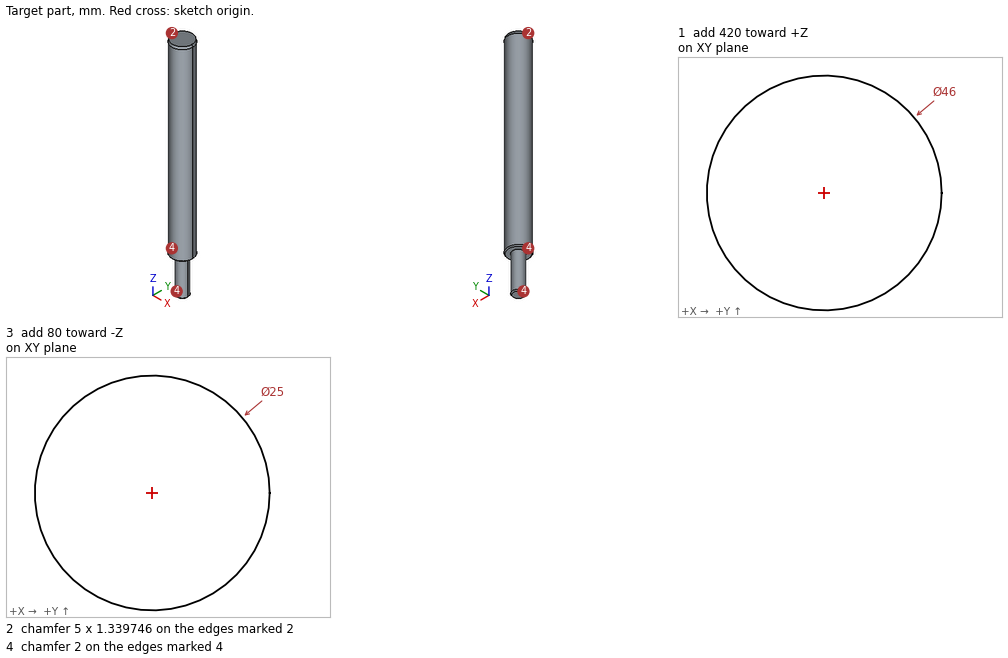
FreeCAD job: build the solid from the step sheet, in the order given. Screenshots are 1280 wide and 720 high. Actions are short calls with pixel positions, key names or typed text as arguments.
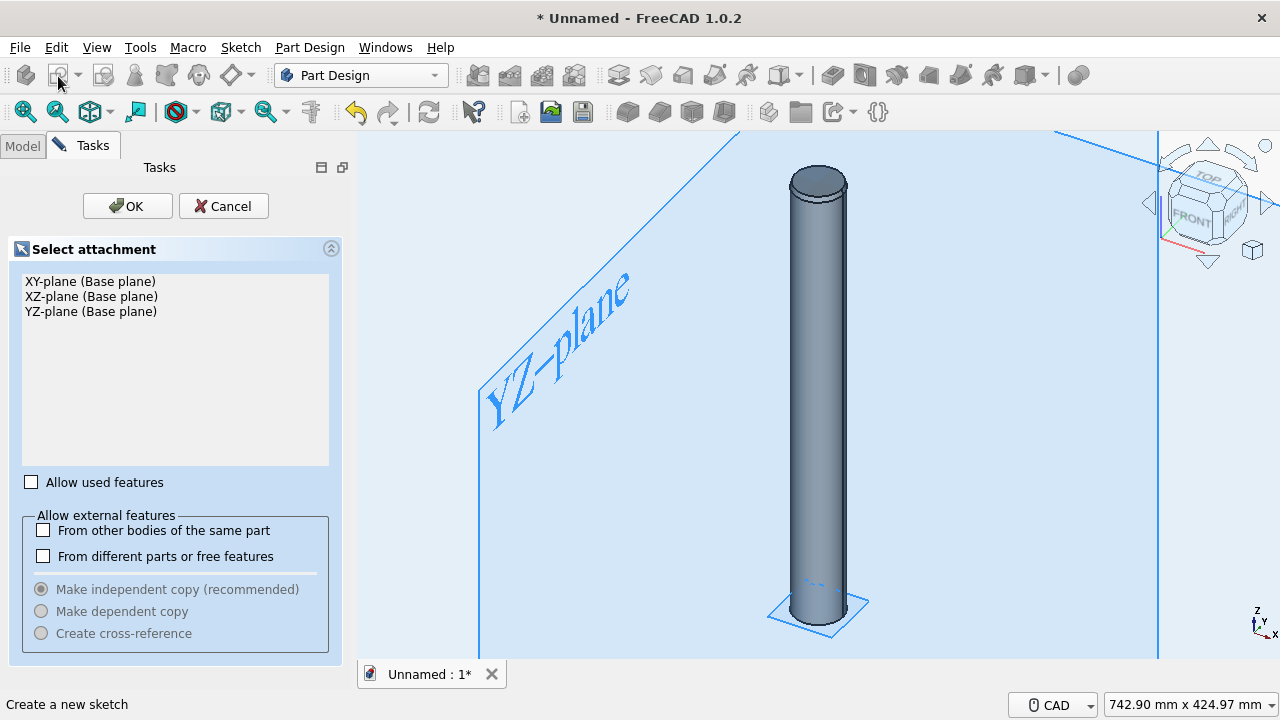
click(82, 282)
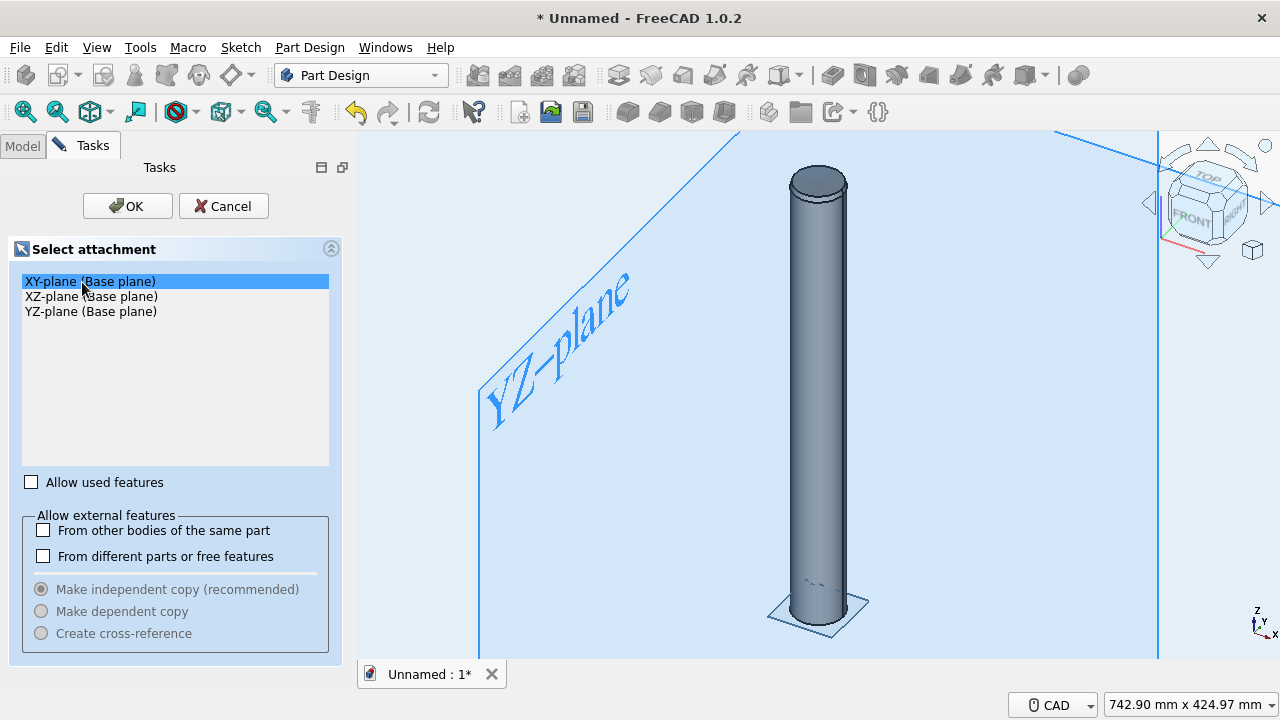
click(128, 206)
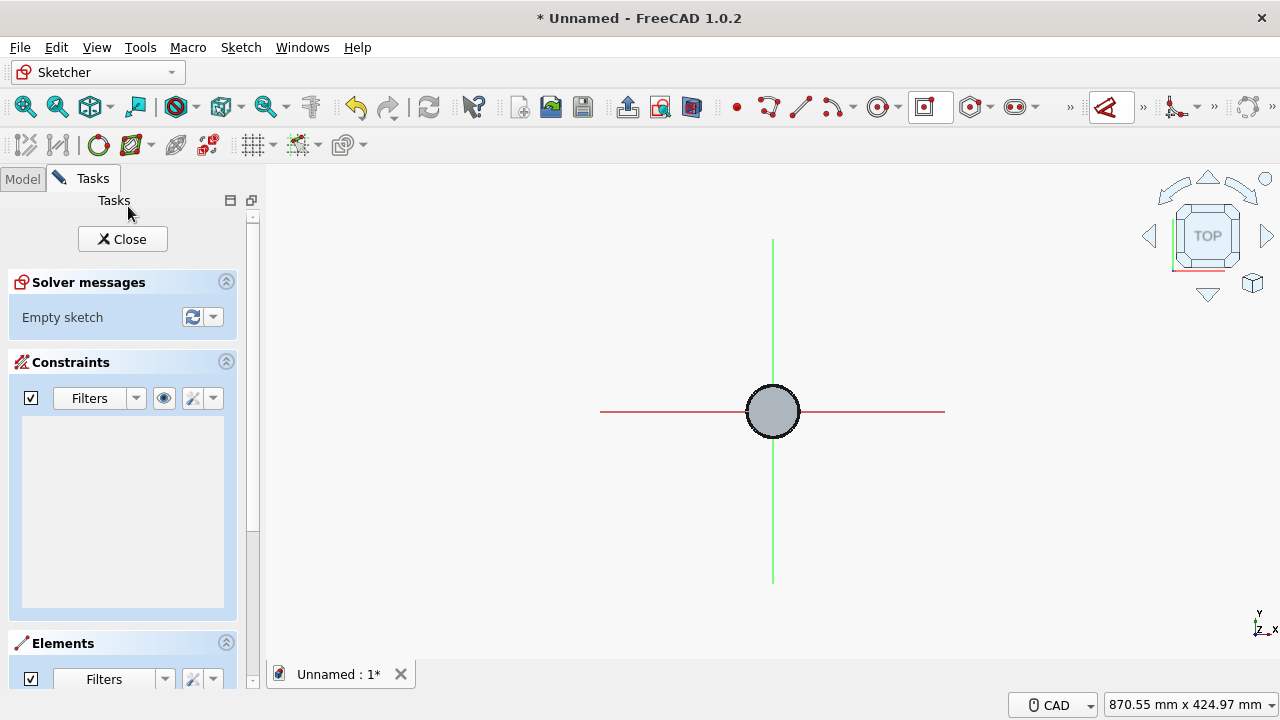
key(q)
key(s)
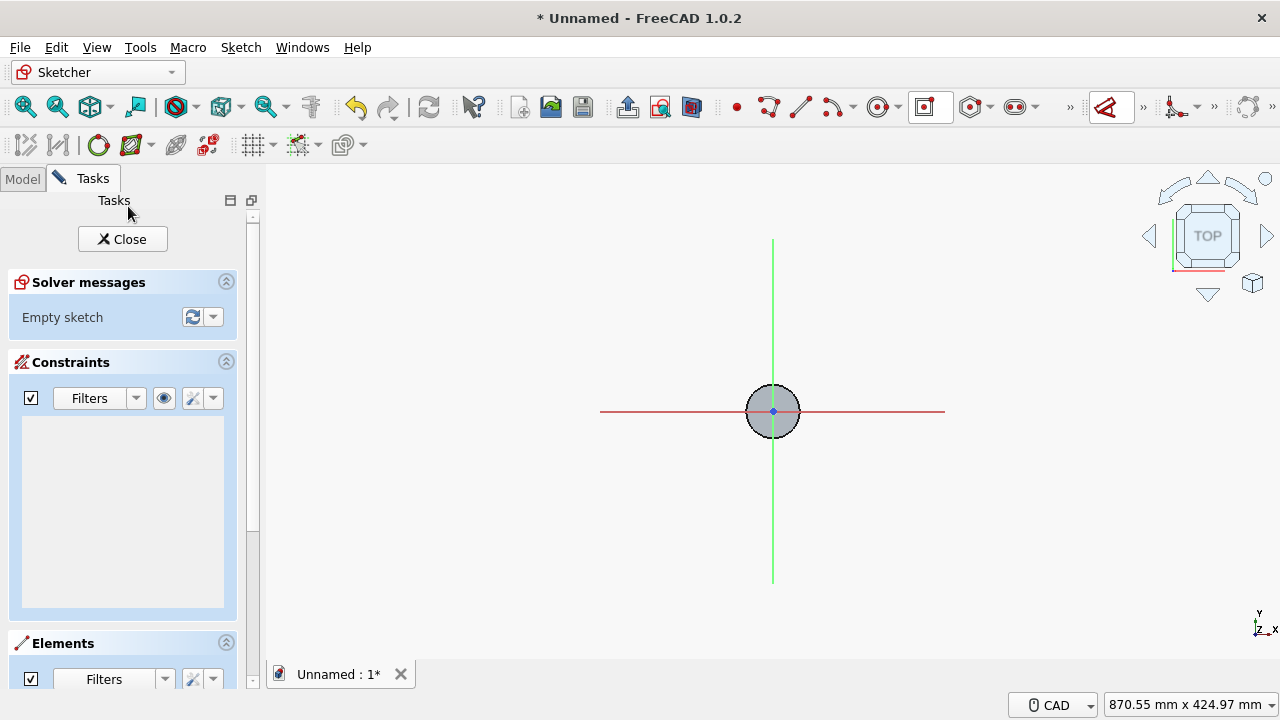
scroll(780, 412, up, 12)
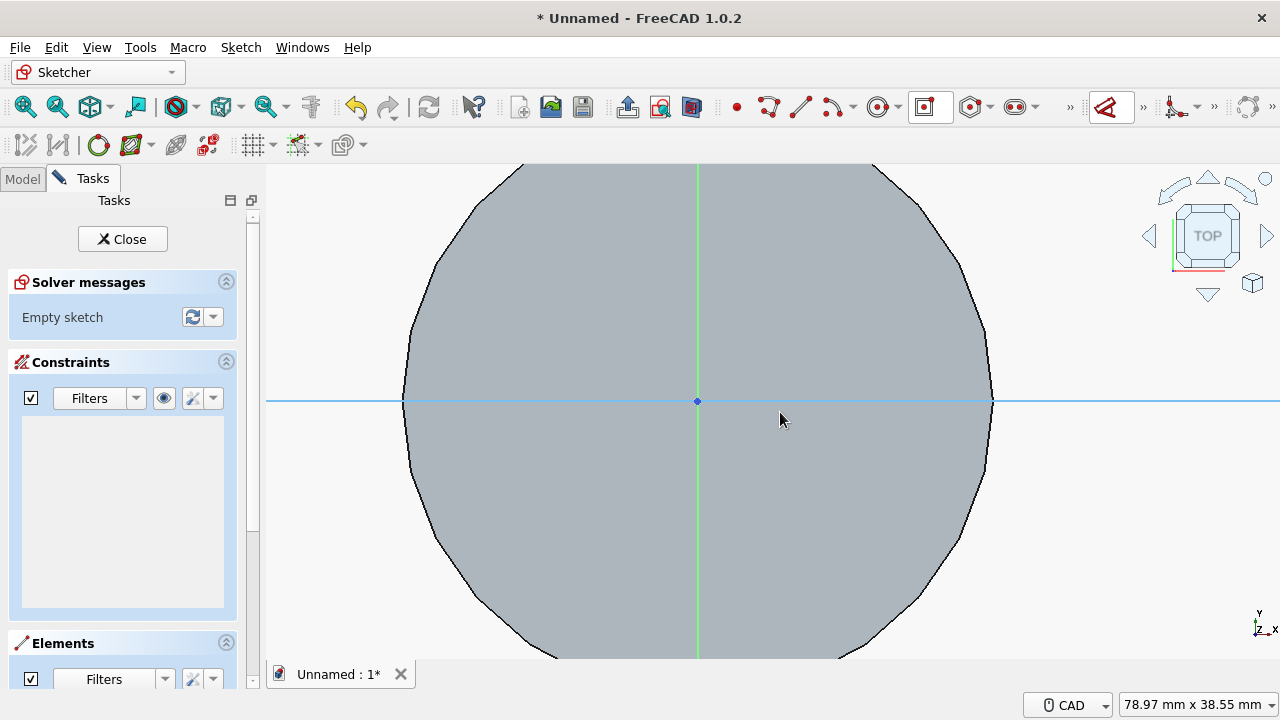
click(878, 108)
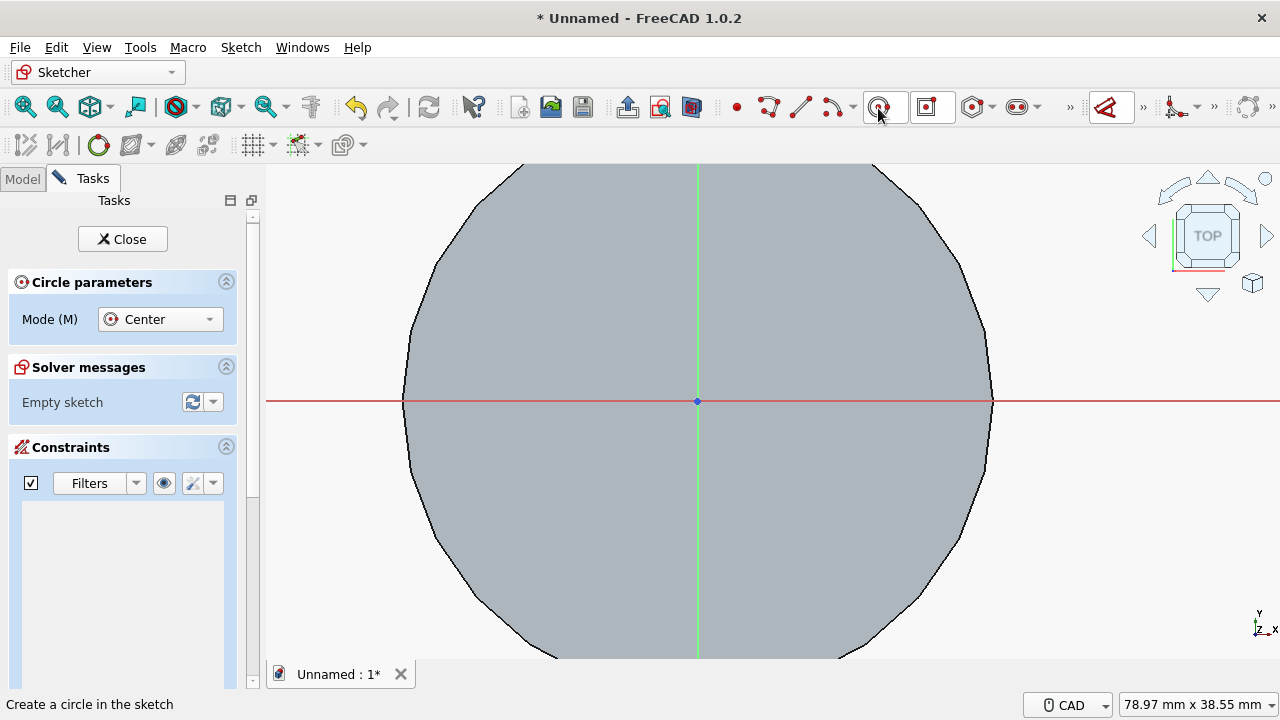
click(698, 401)
move(811, 288)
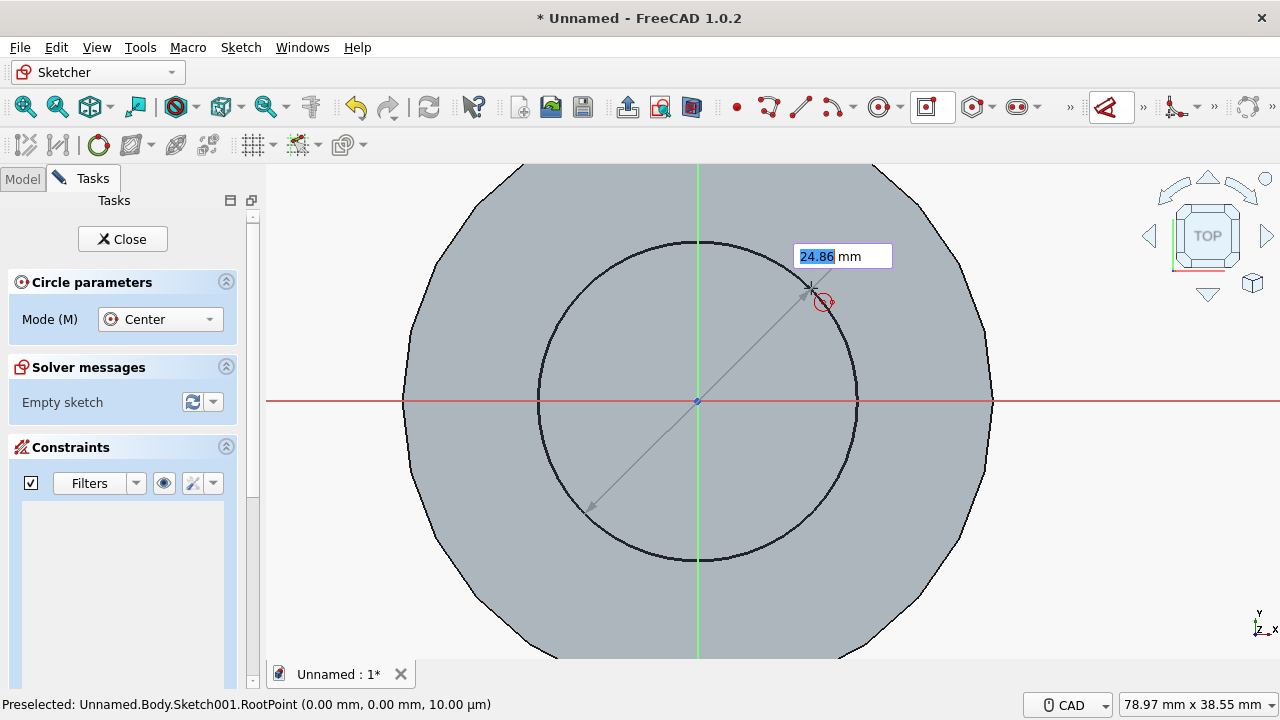
text(25)
key(Return)
key(Escape)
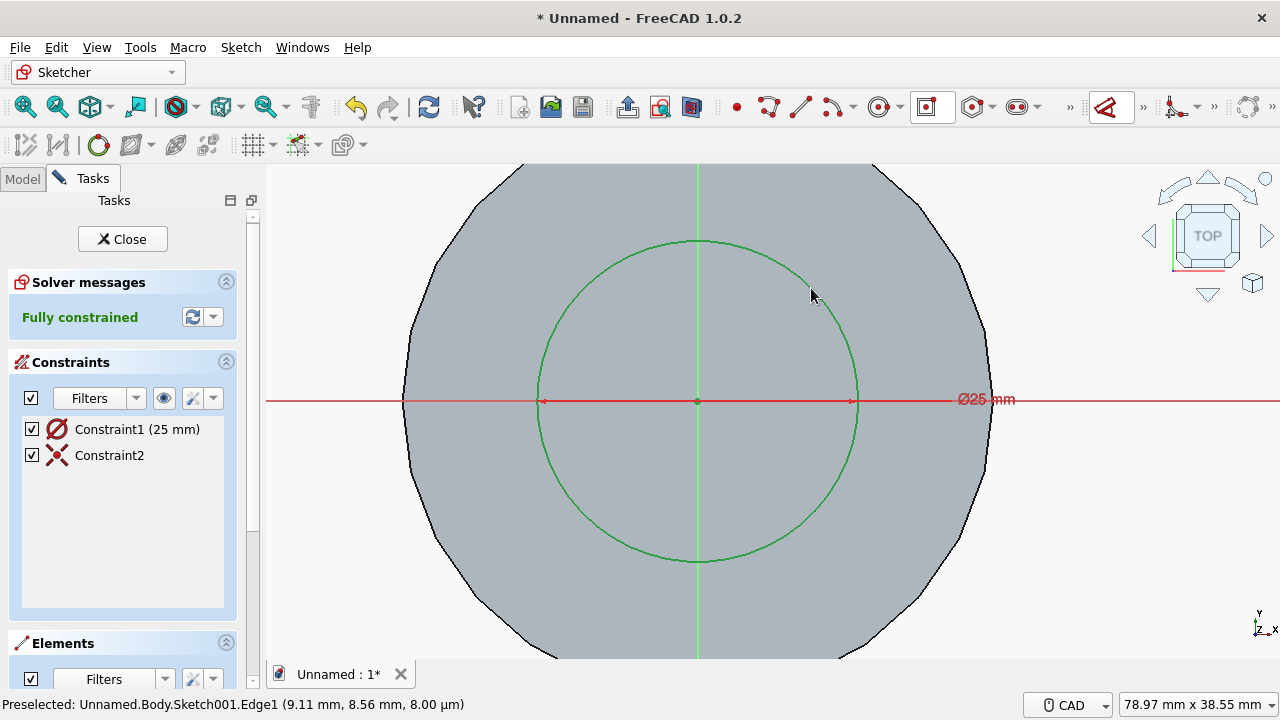
click(123, 239)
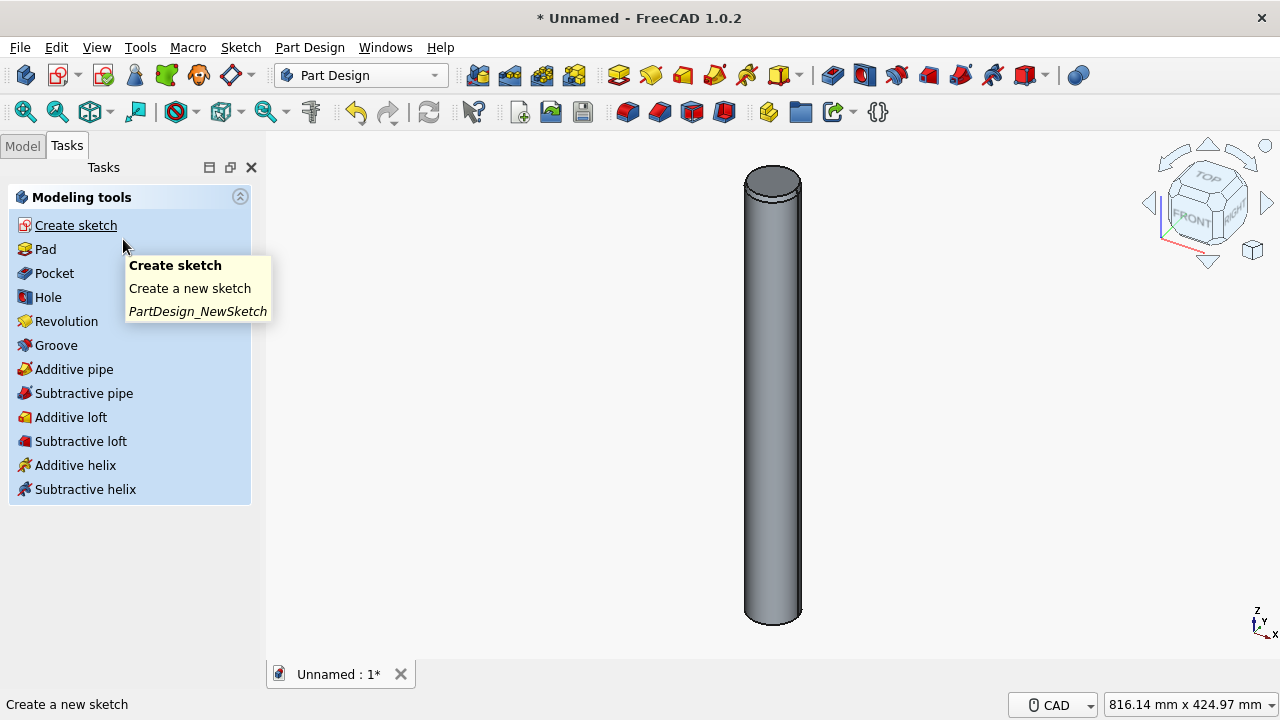
click(620, 76)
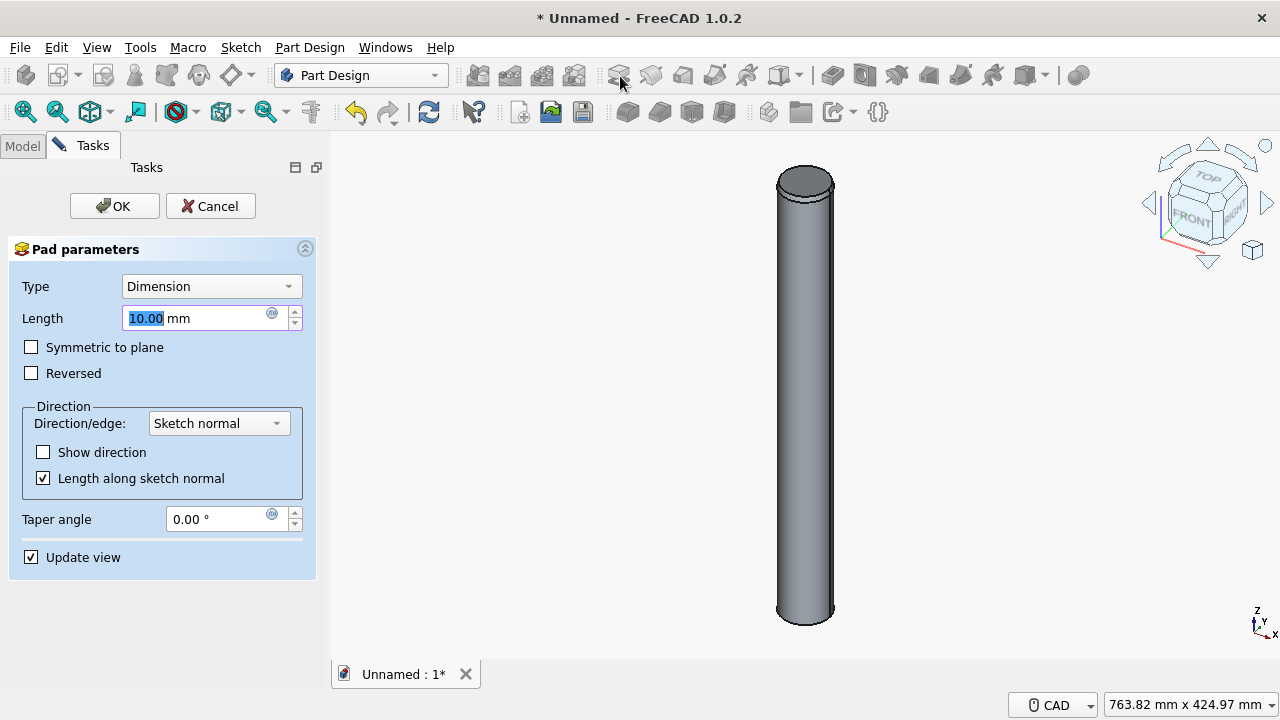
text(80)
key(Tab)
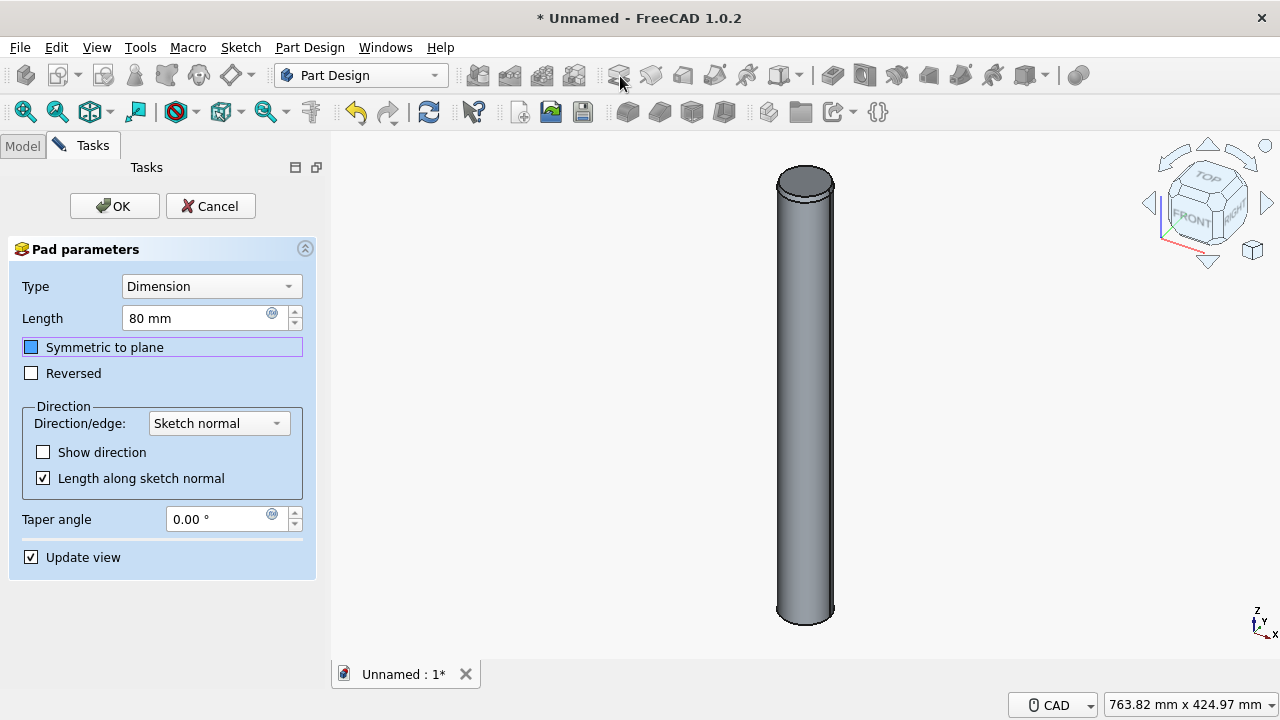
click(30, 373)